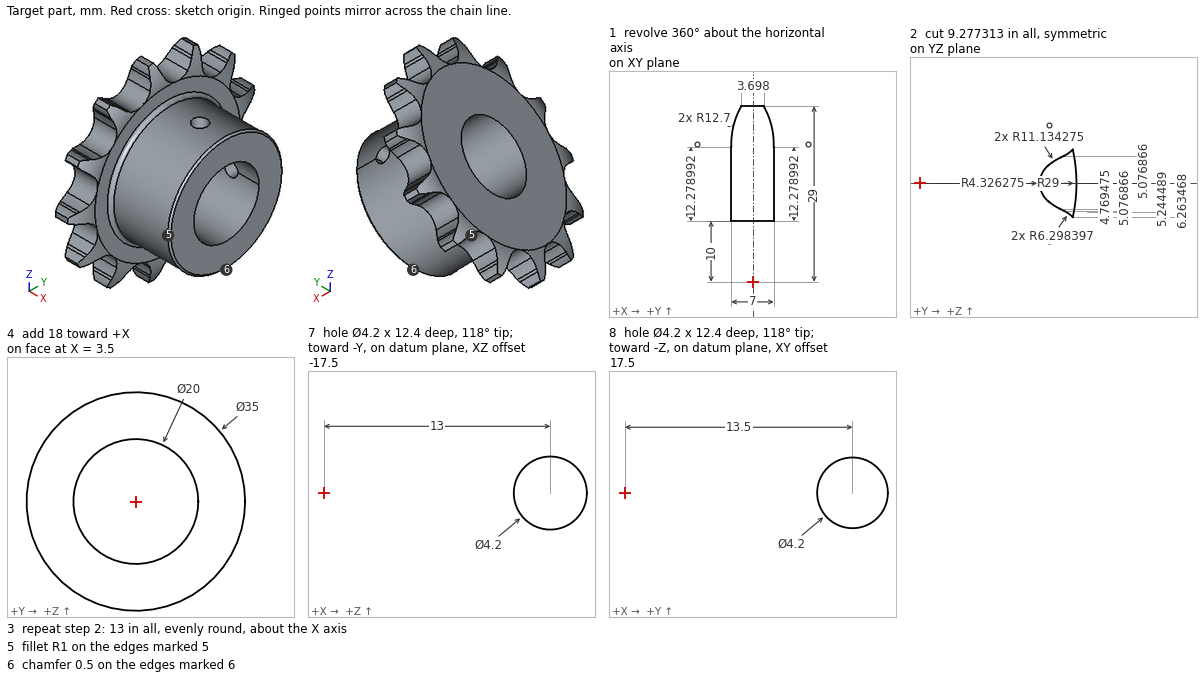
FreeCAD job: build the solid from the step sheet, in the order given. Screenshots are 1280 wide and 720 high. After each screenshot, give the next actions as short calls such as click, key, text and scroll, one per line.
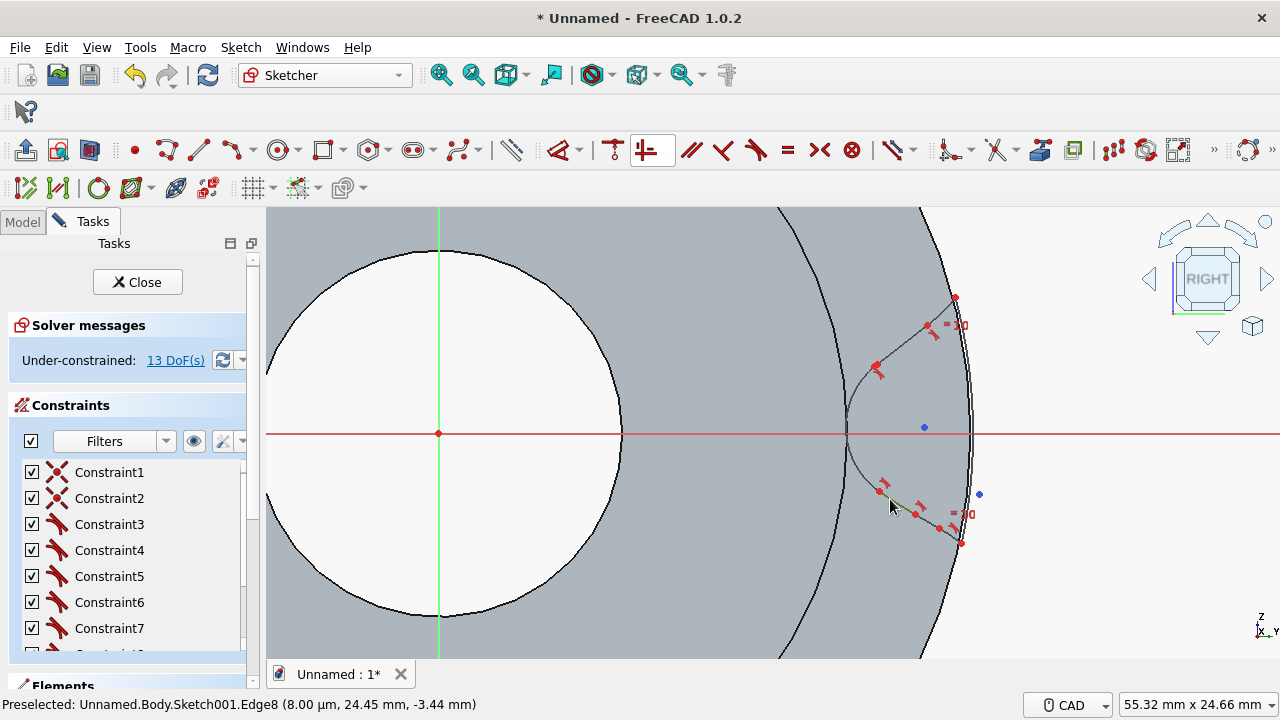
click(788, 150)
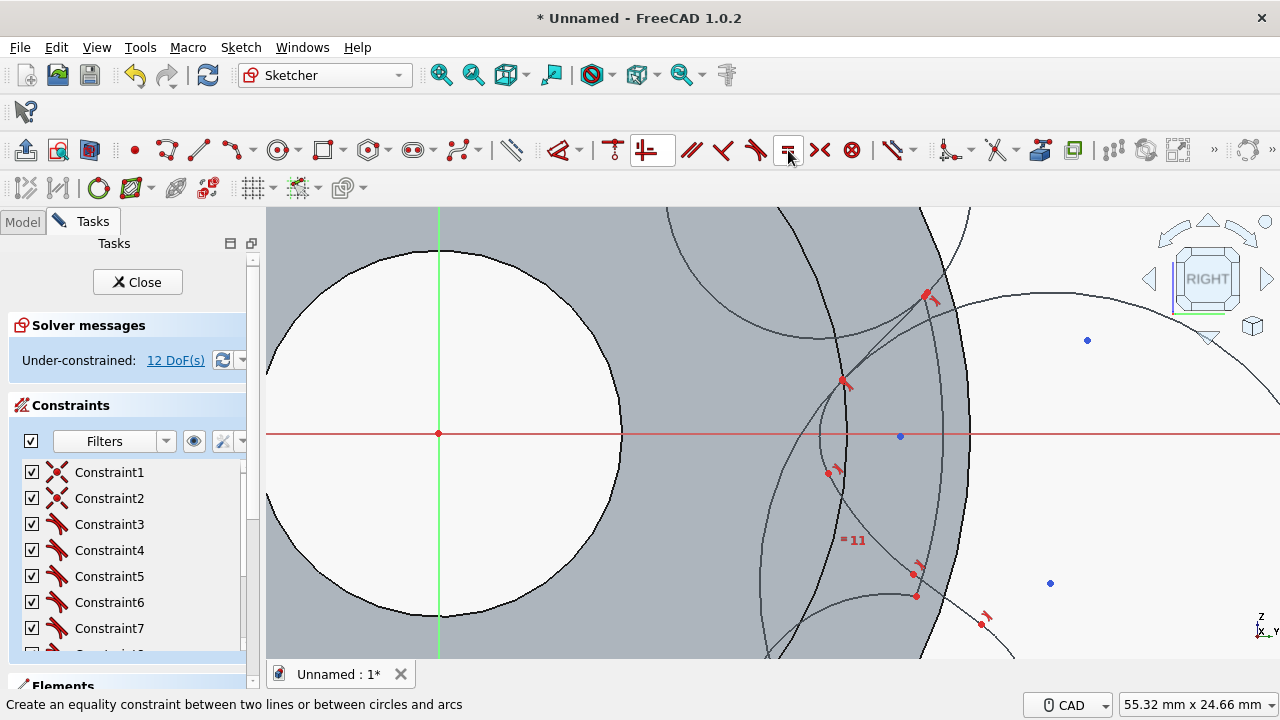
click(901, 437)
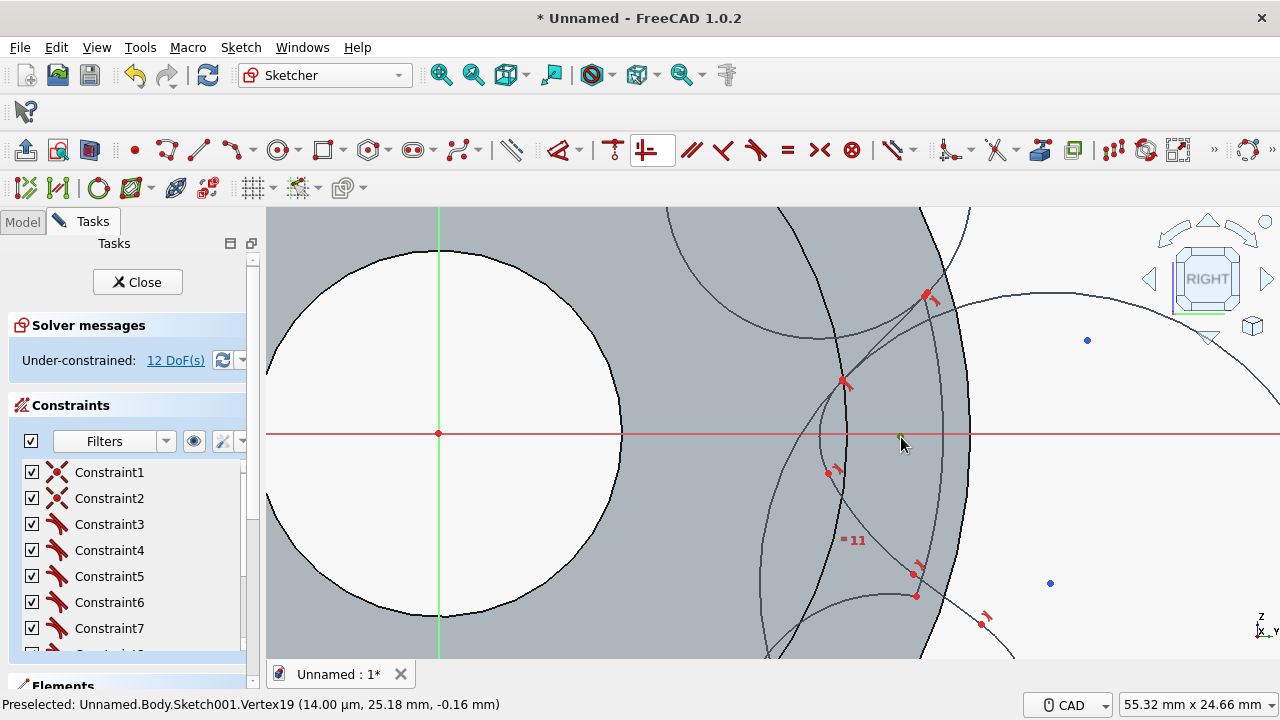
click(353, 434)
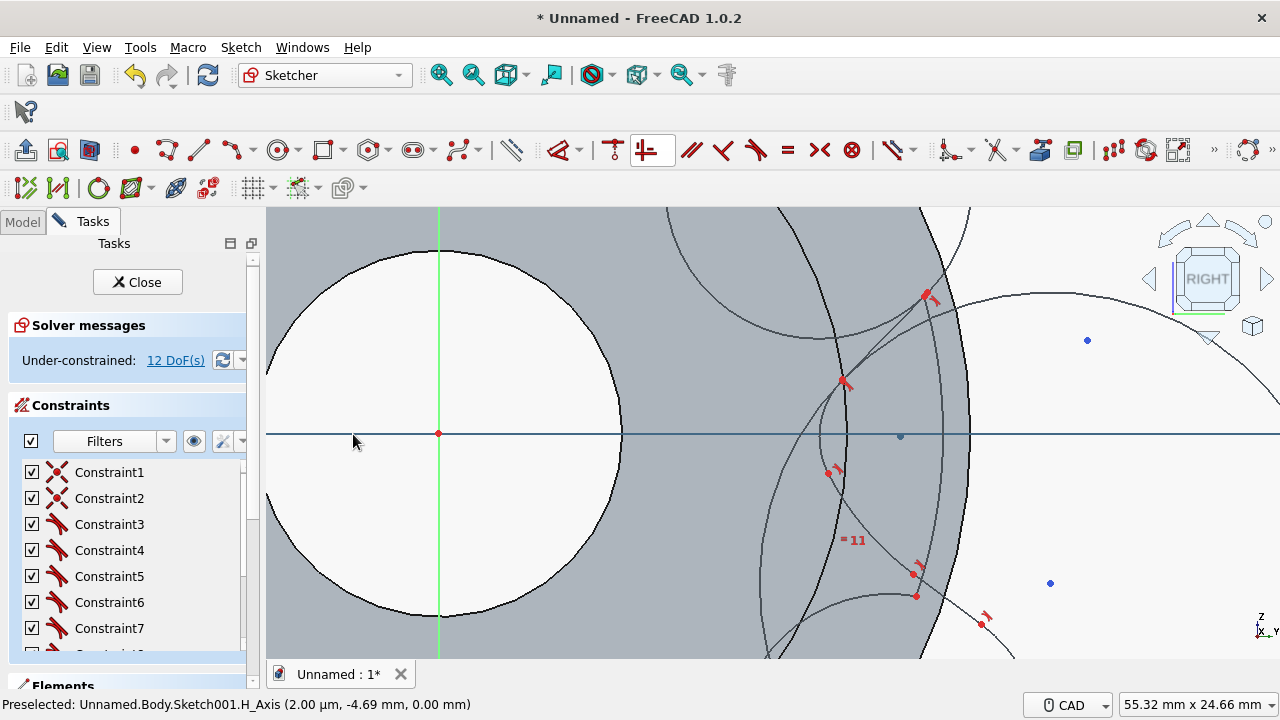
click(614, 150)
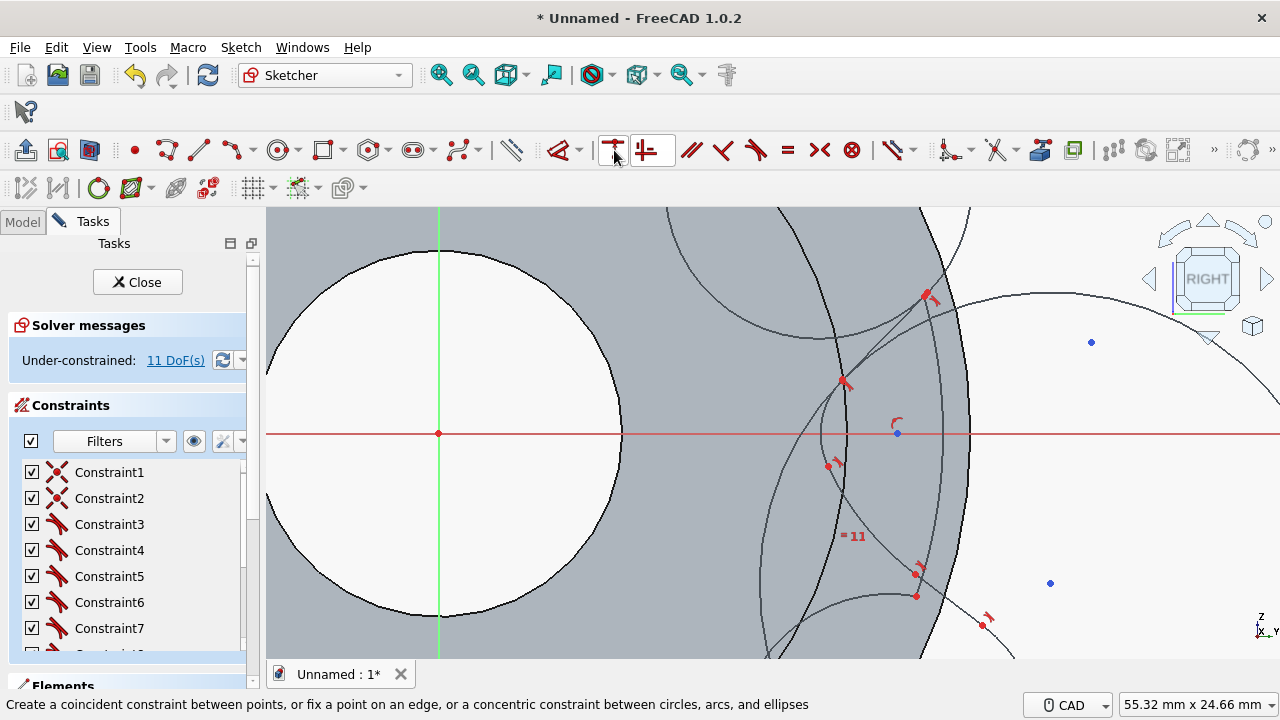
scroll(704, 235, down, 2)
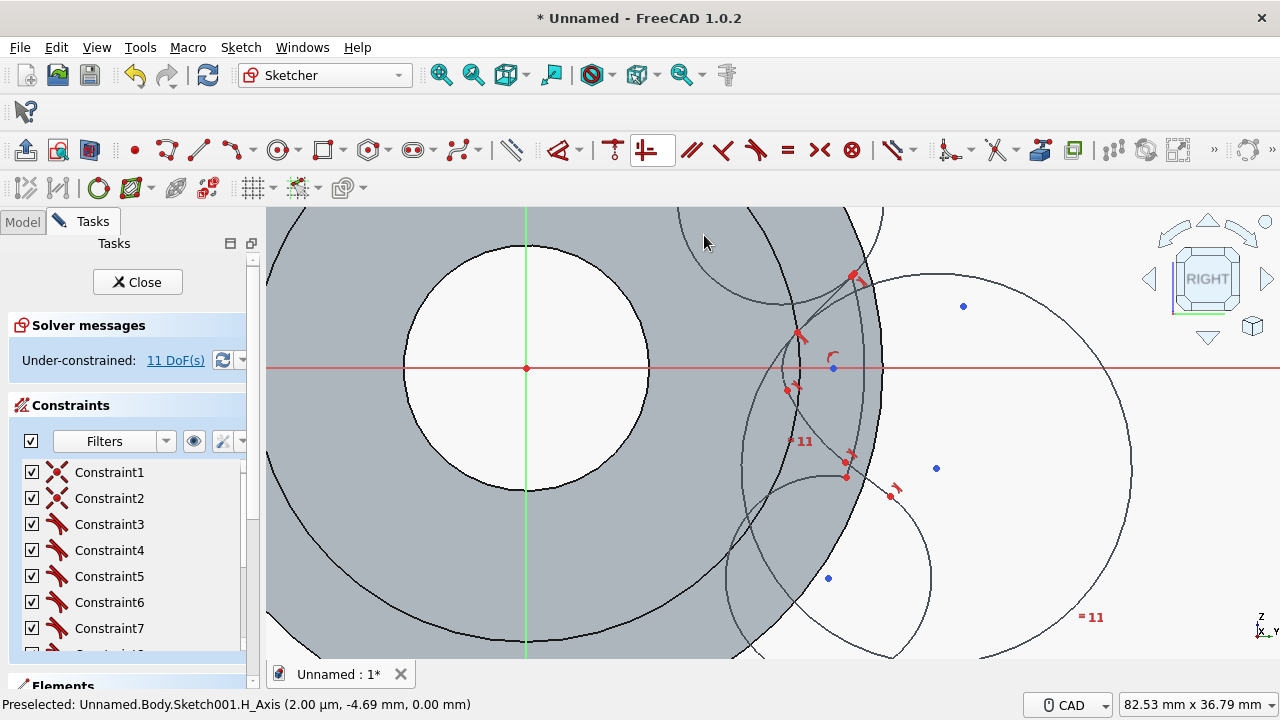
click(829, 578)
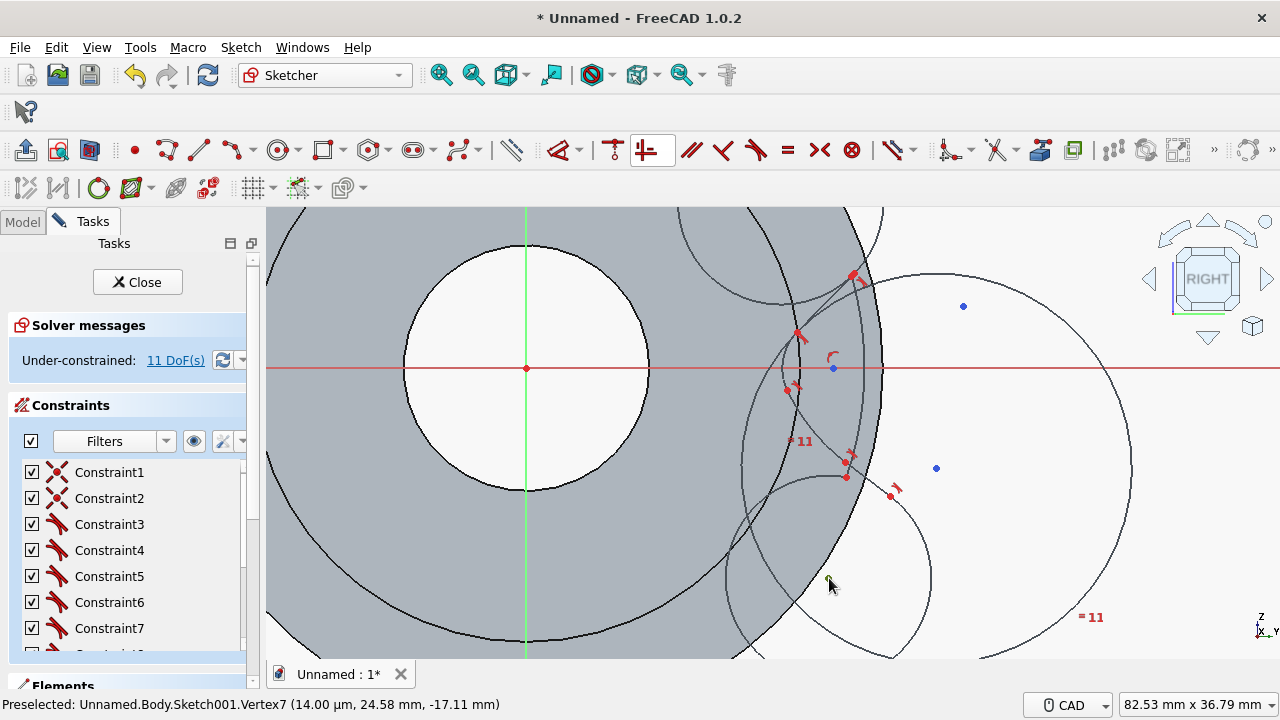
scroll(705, 236, up, 2)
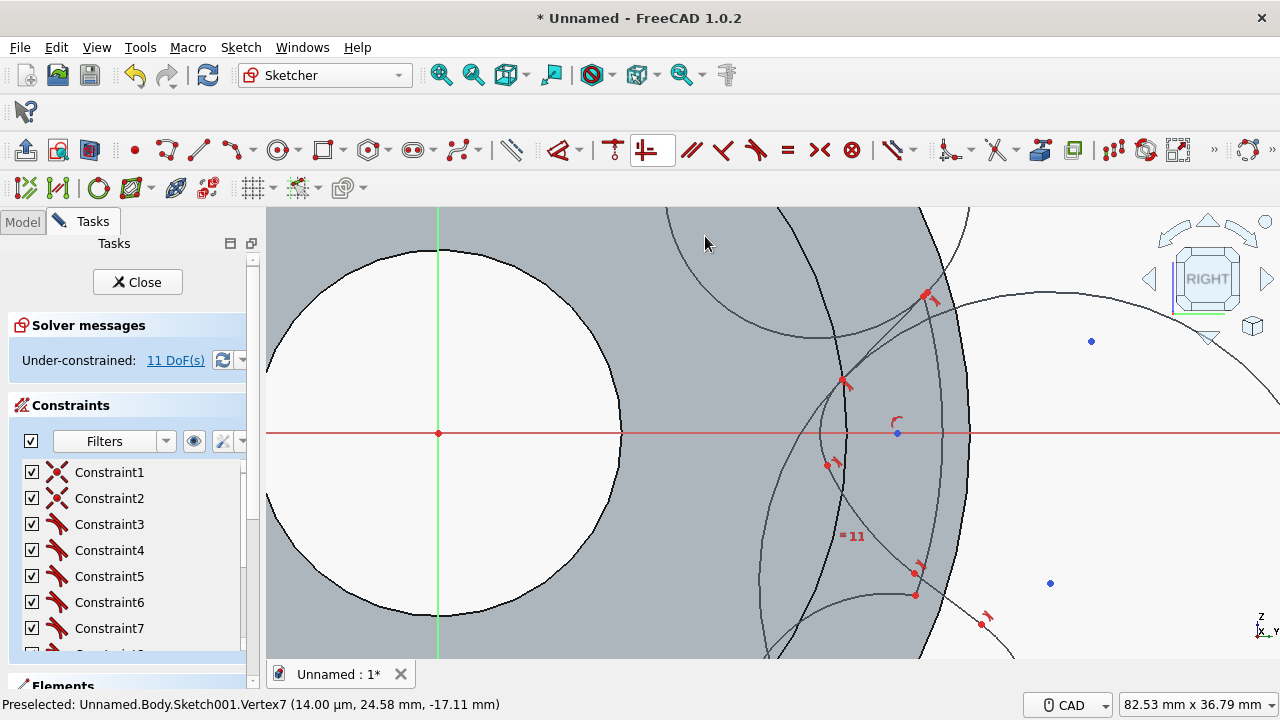
scroll(706, 631, down, 1)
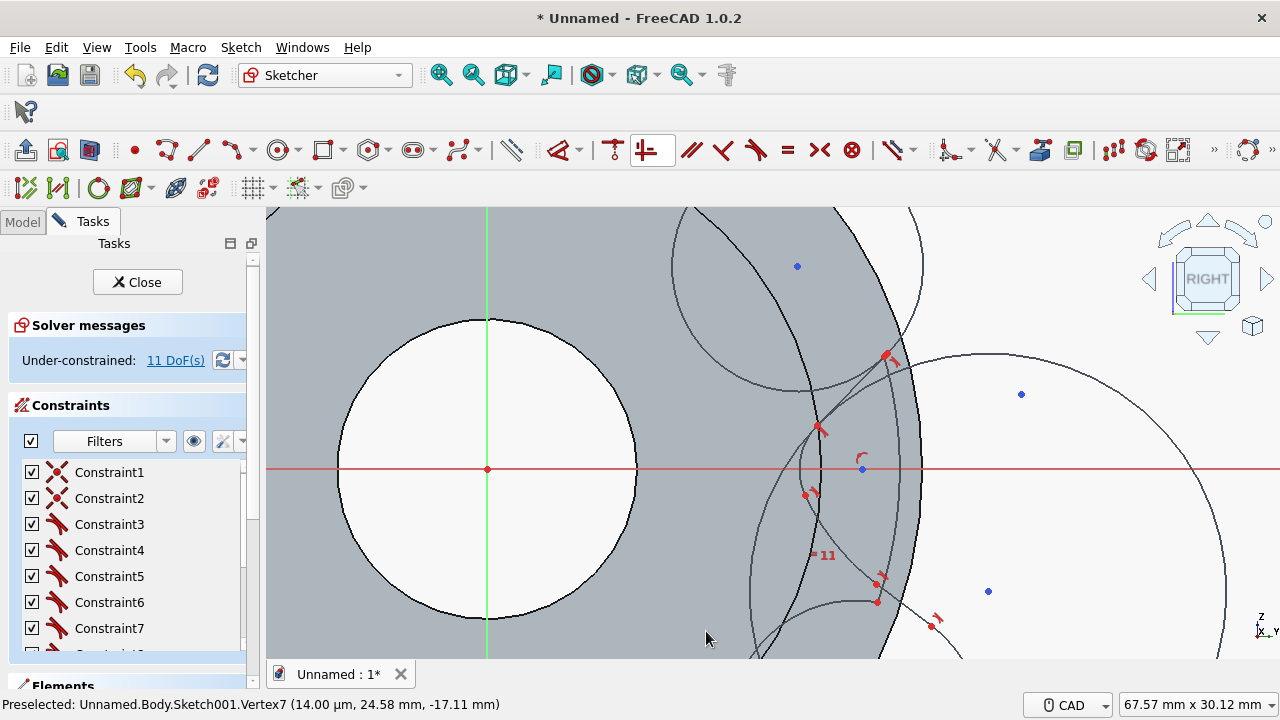
click(798, 266)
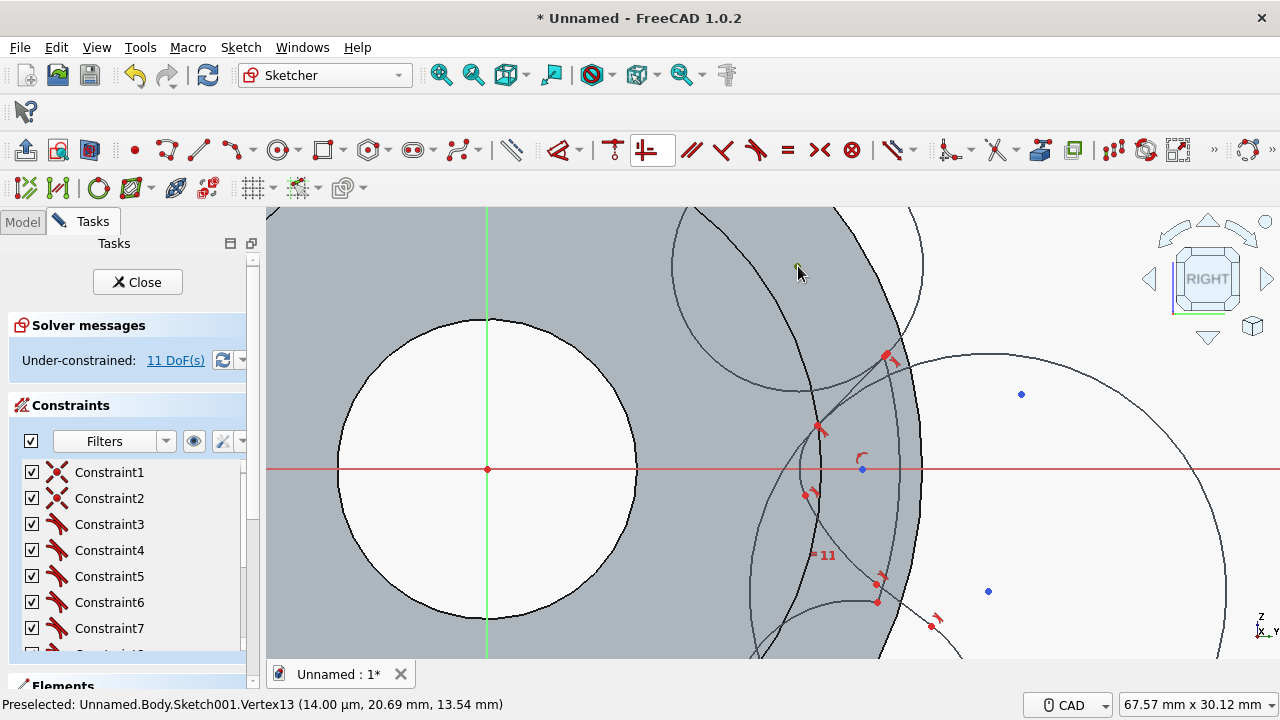
click(353, 469)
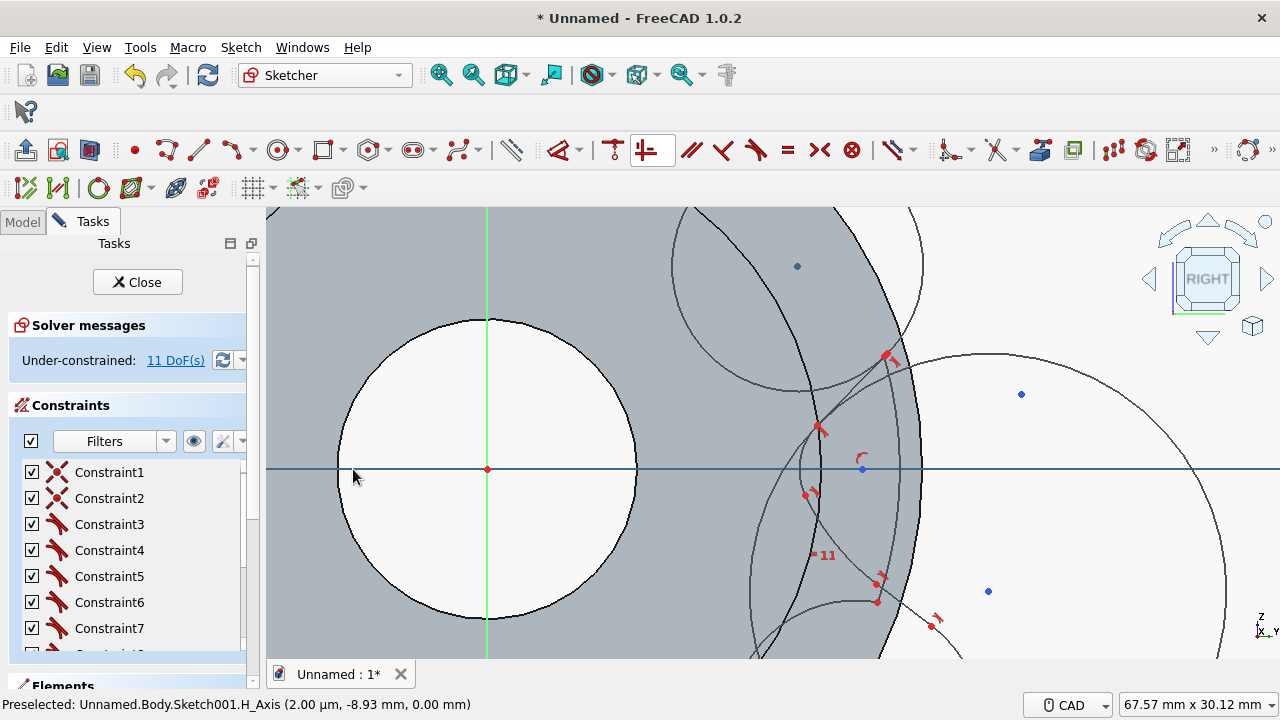
click(820, 150)